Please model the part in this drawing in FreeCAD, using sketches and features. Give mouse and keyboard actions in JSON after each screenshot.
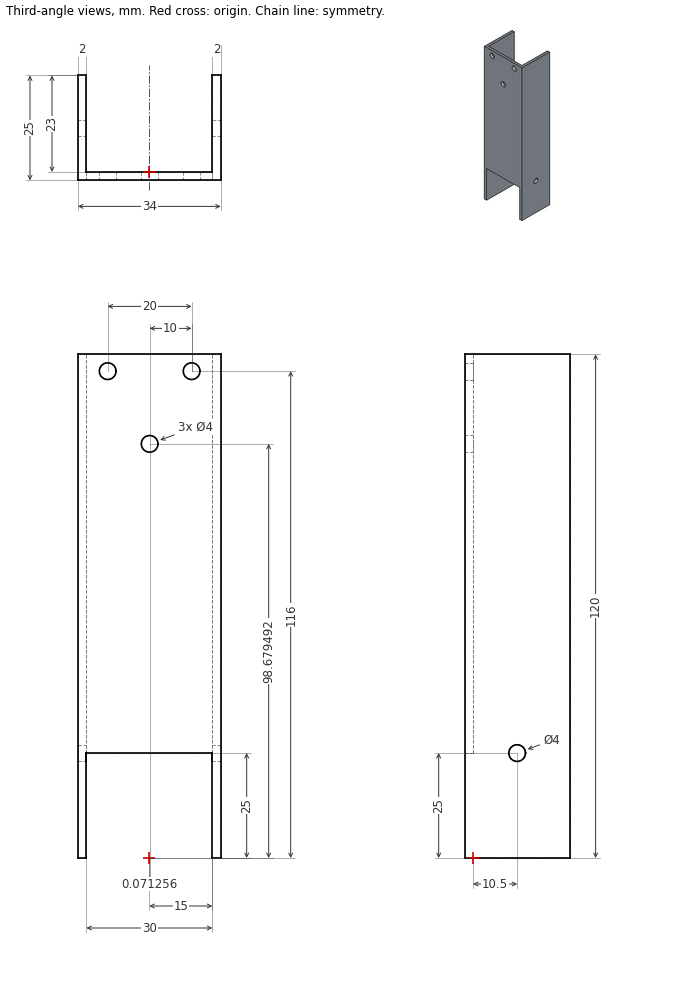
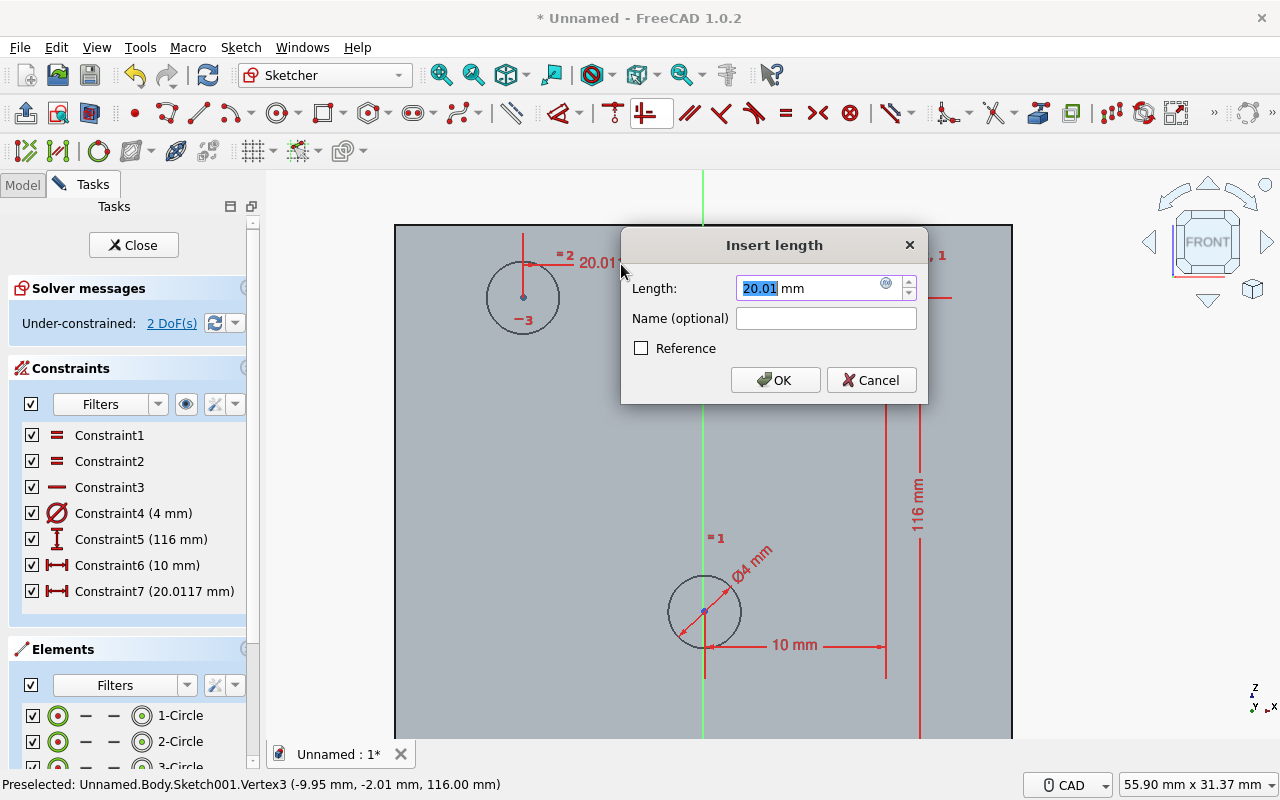
{"action": "type", "text": "20"}
{"action": "key", "text": "Return"}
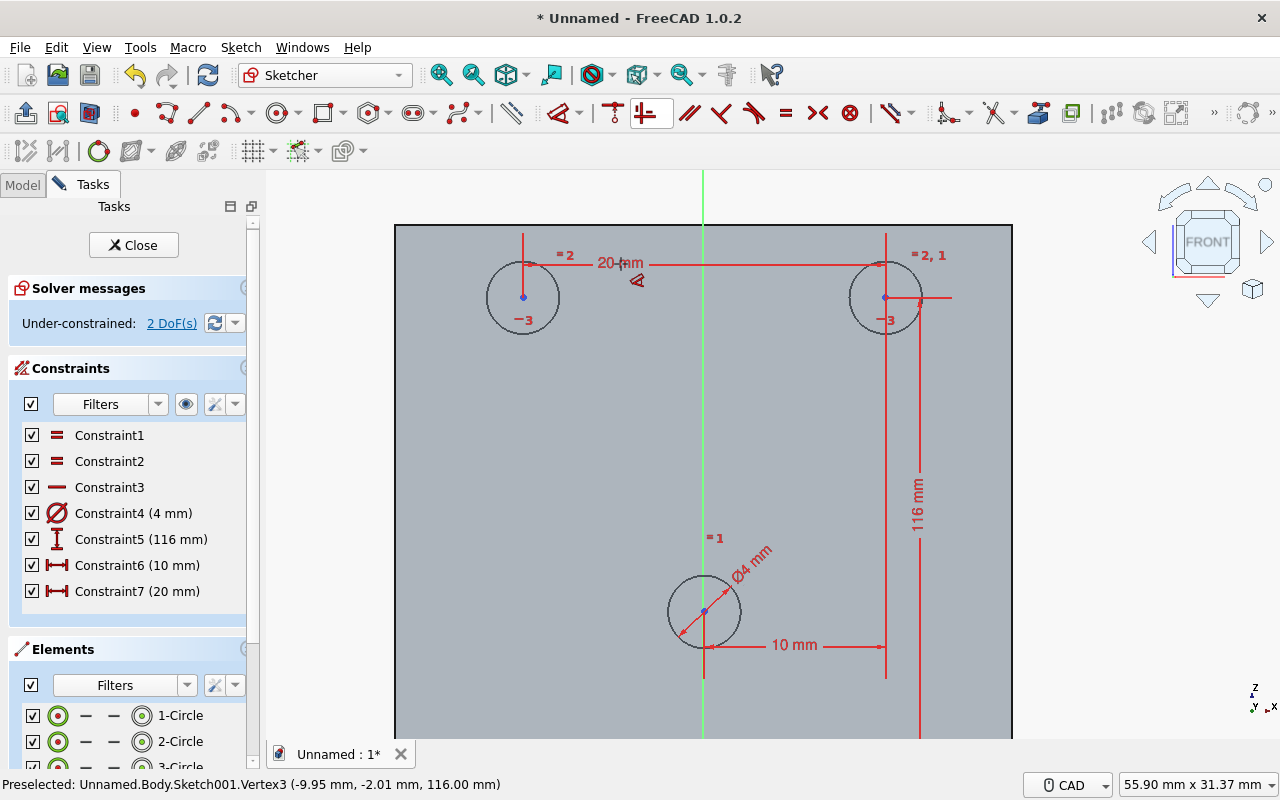
{"action": "scroll", "coordinate": [704, 612], "scroll_direction": "up", "scroll_amount": 18}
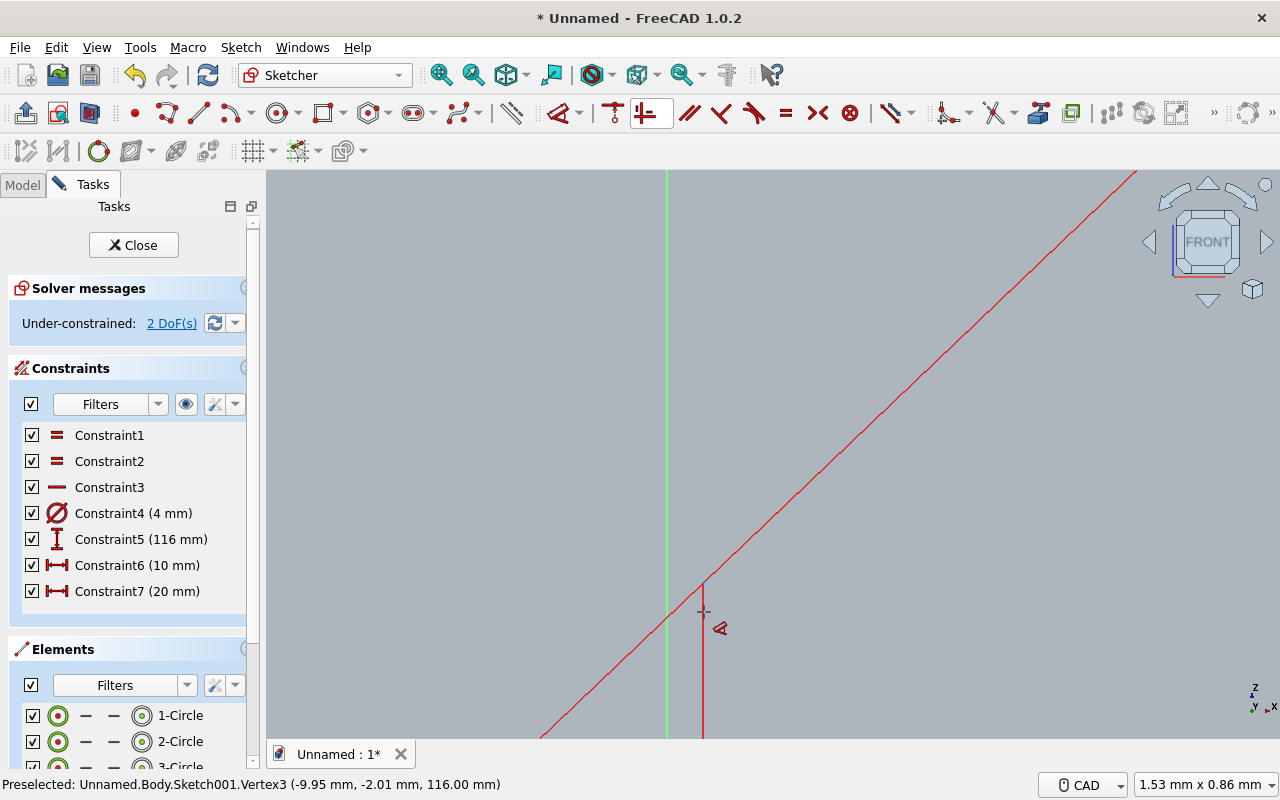
{"action": "left_click", "coordinate": [703, 583]}
{"action": "left_click", "coordinate": [685, 549]}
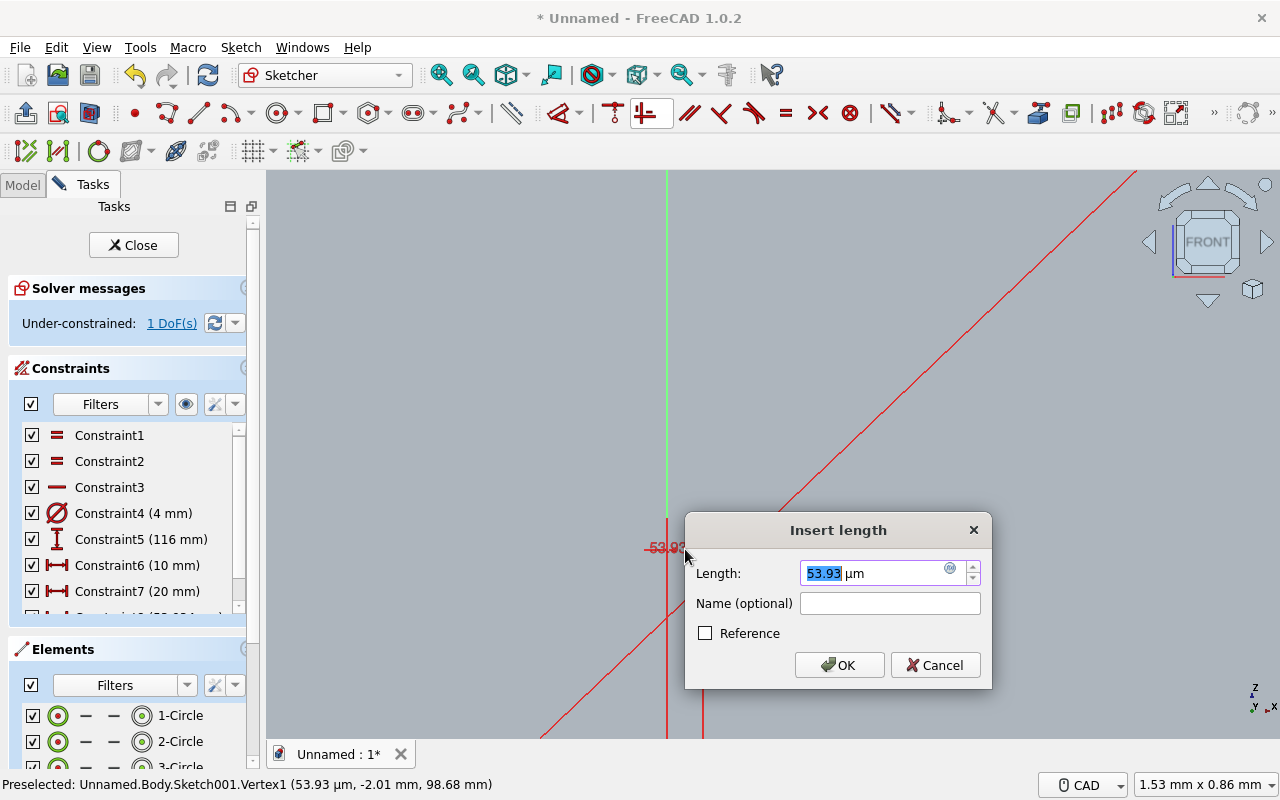
{"action": "key", "text": "ctrl+a"}
{"action": "type", "text": "0.071256 mm"}
{"action": "key", "text": "Return"}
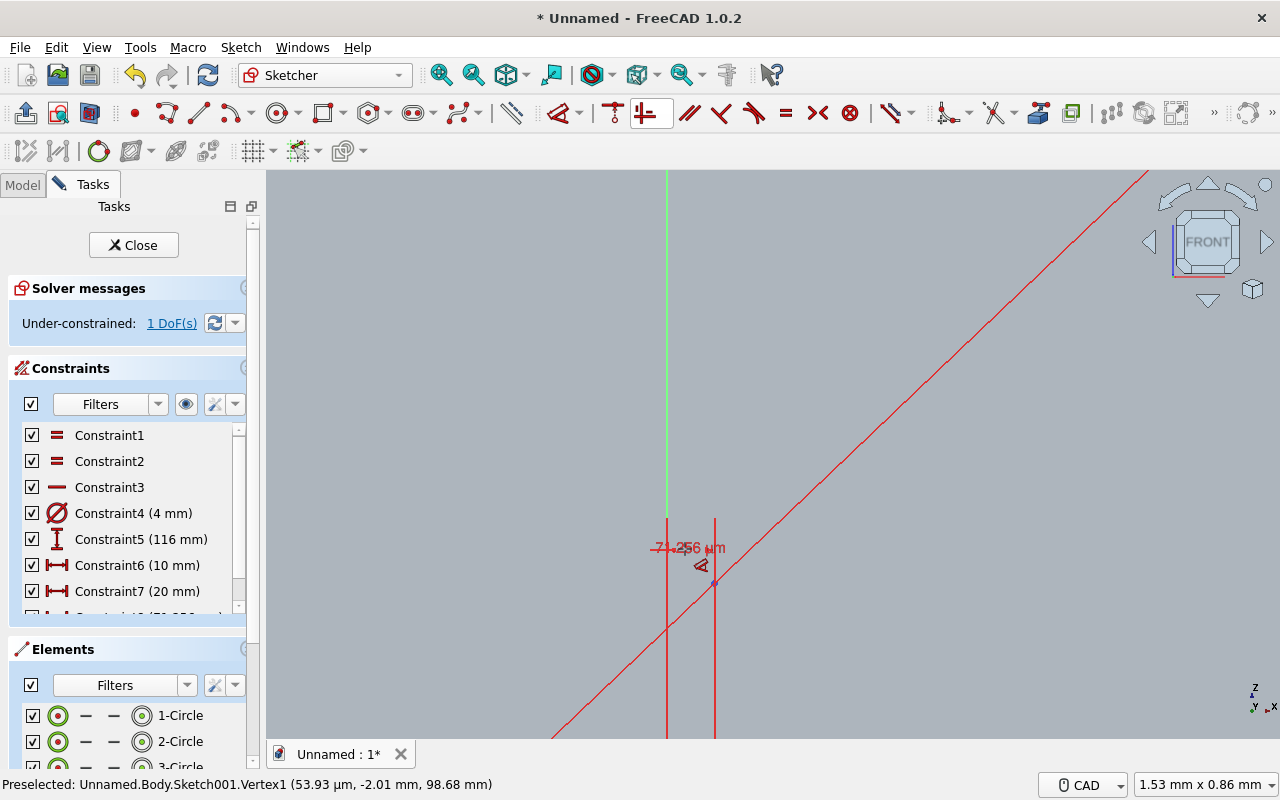
{"action": "scroll", "coordinate": [704, 612], "scroll_direction": "down", "scroll_amount": 18}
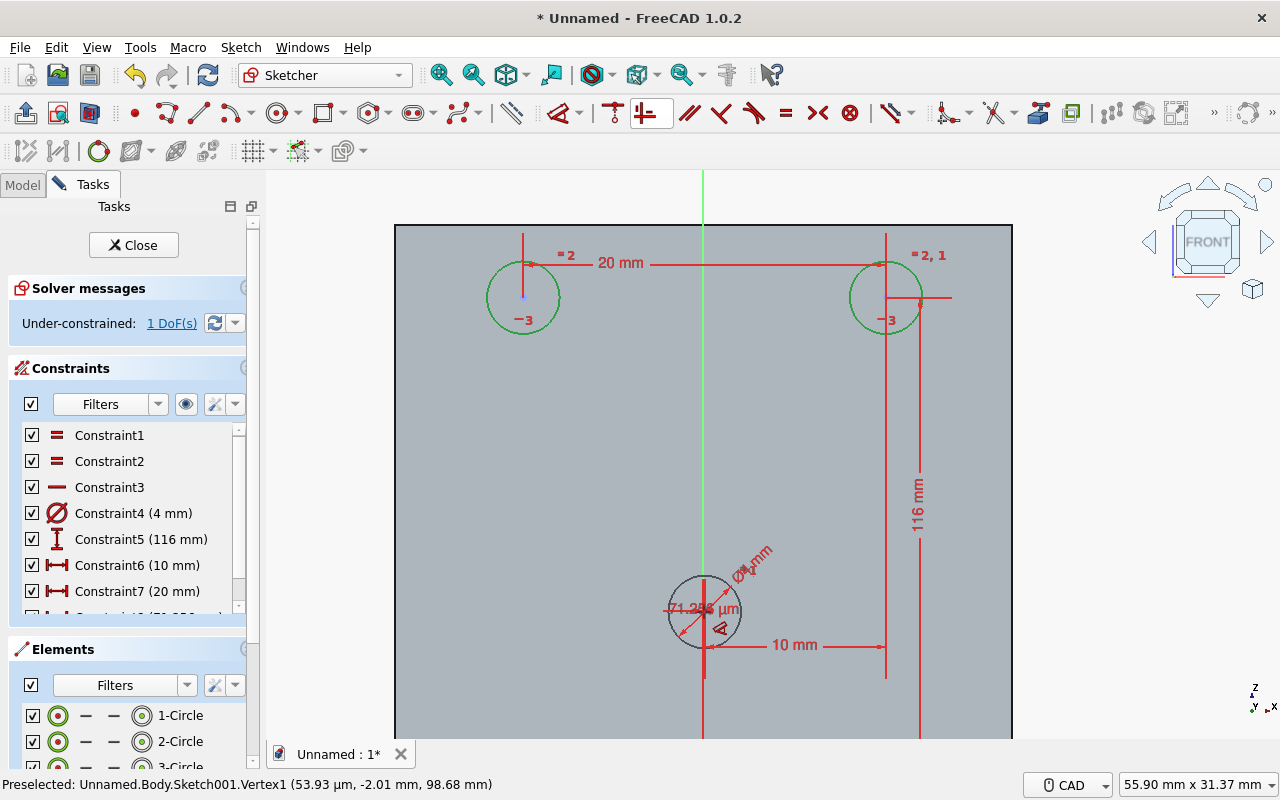
{"action": "left_click", "coordinate": [705, 612]}
{"action": "left_click", "coordinate": [669, 661]}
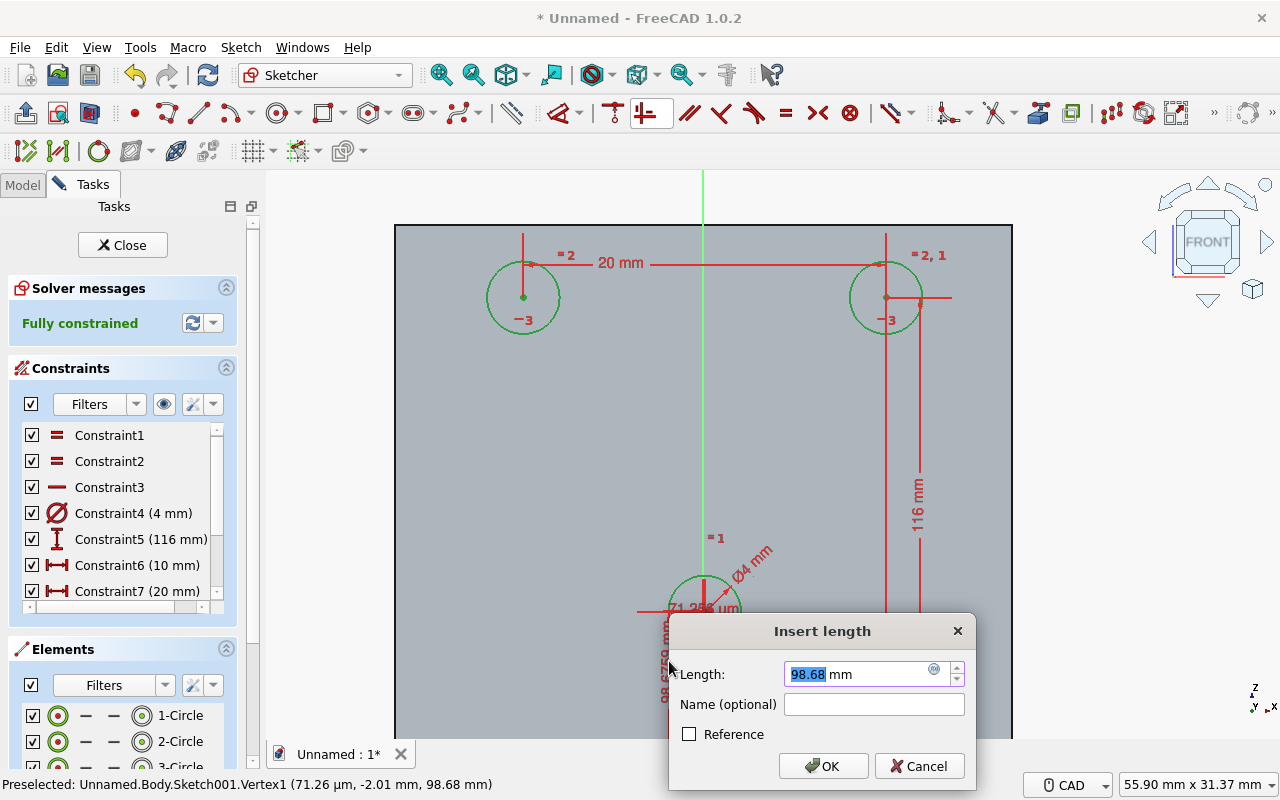
{"action": "type", "text": "98.679492"}
{"action": "key", "text": "Return"}
{"action": "key", "text": "Escape"}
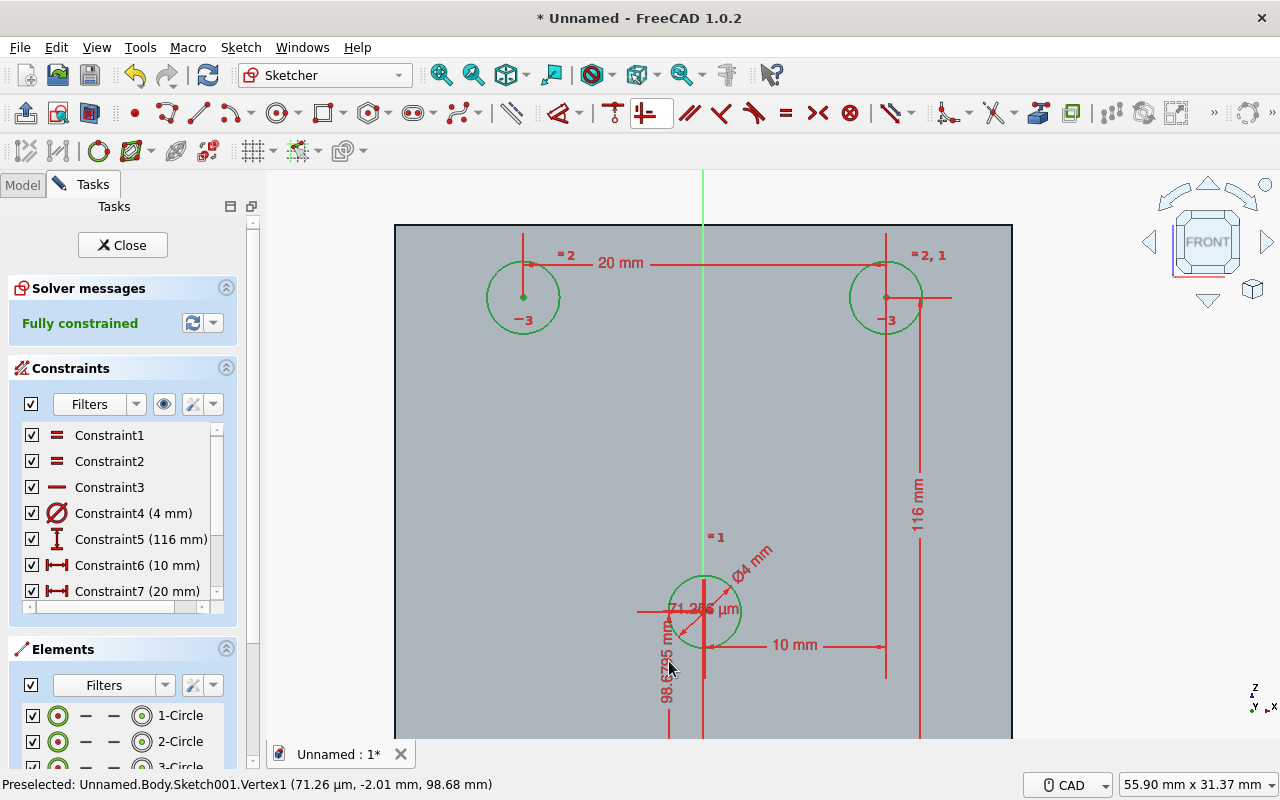
{"action": "left_click", "coordinate": [123, 245]}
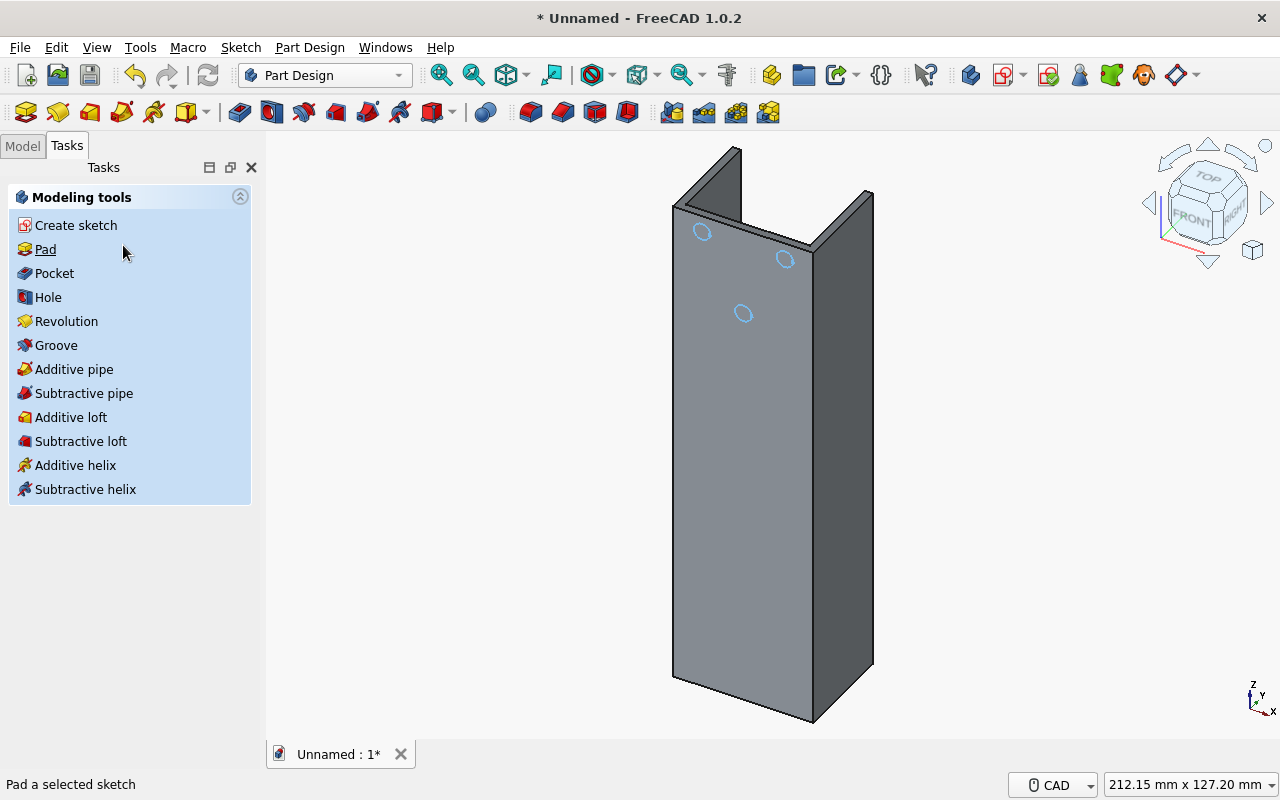
{"action": "left_click", "coordinate": [240, 112]}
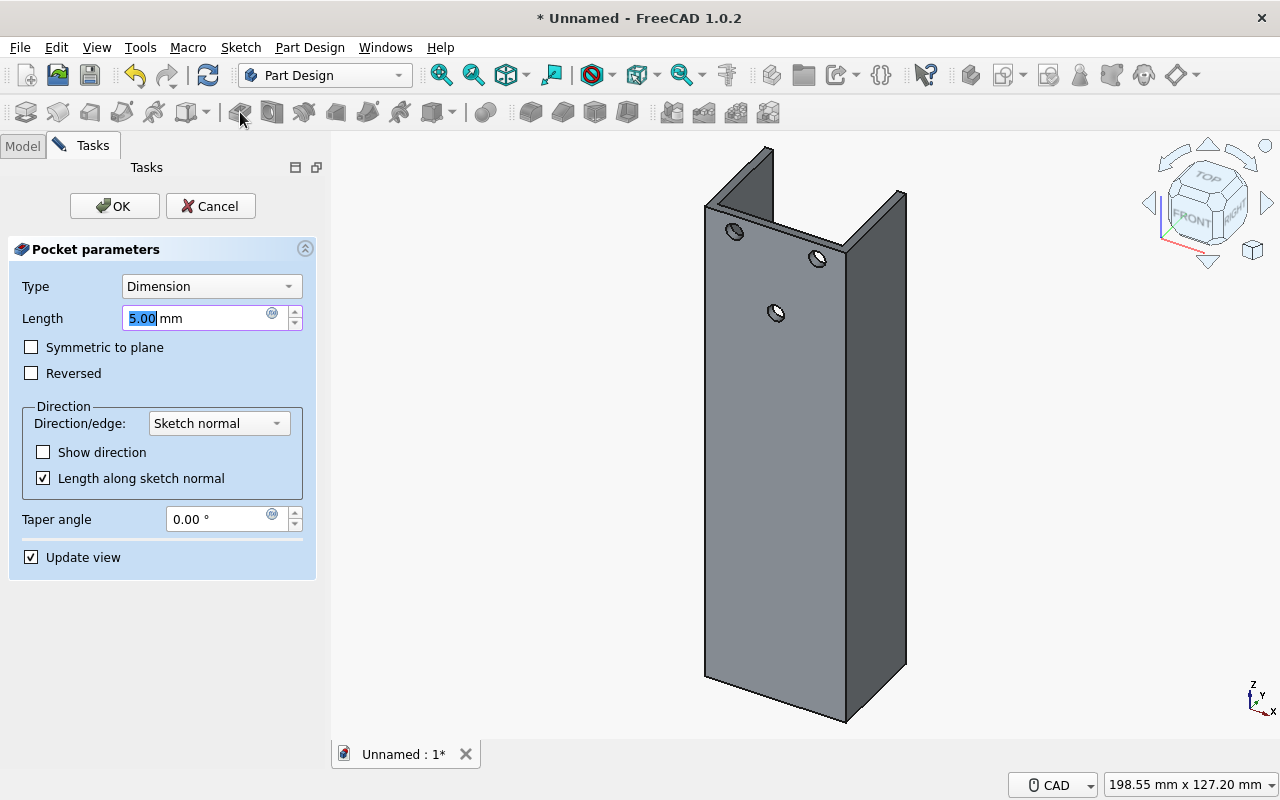
{"action": "left_click", "coordinate": [212, 286]}